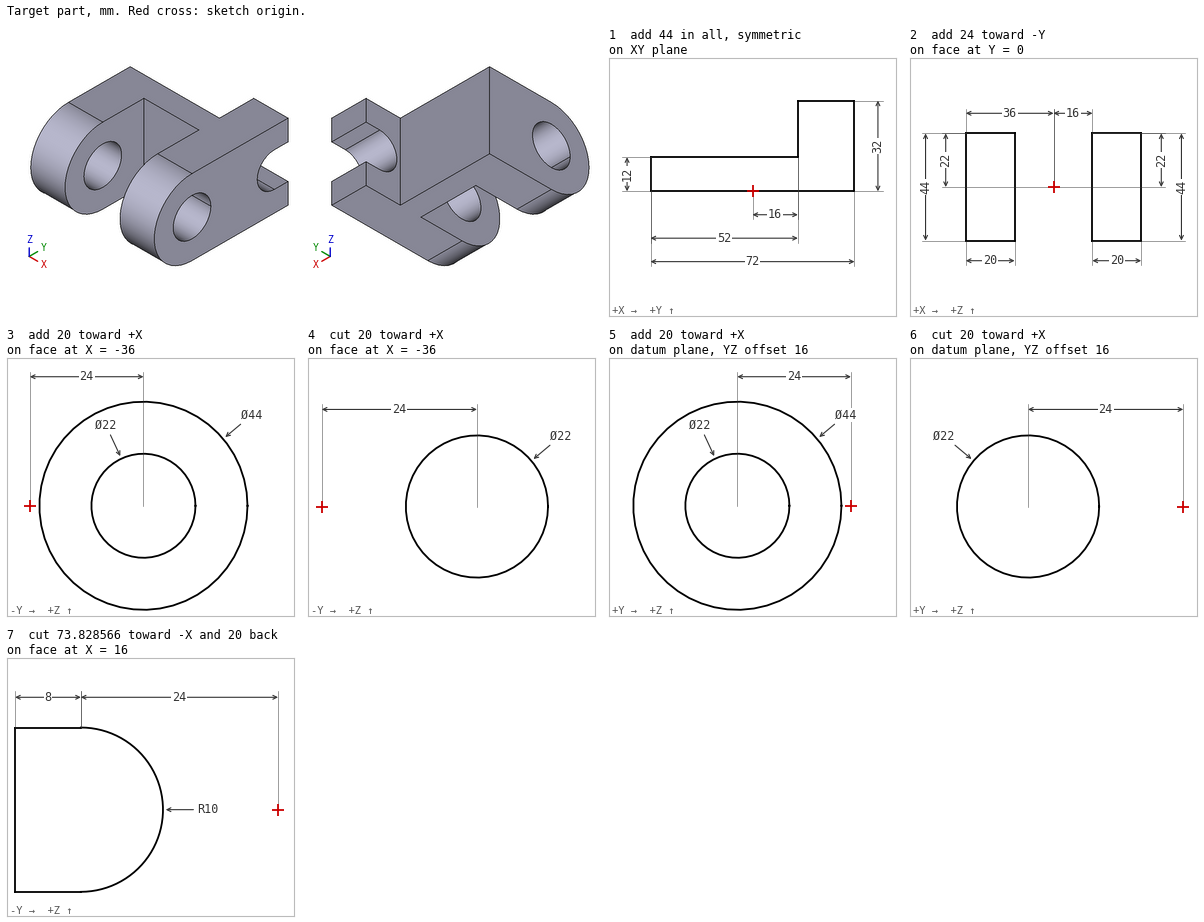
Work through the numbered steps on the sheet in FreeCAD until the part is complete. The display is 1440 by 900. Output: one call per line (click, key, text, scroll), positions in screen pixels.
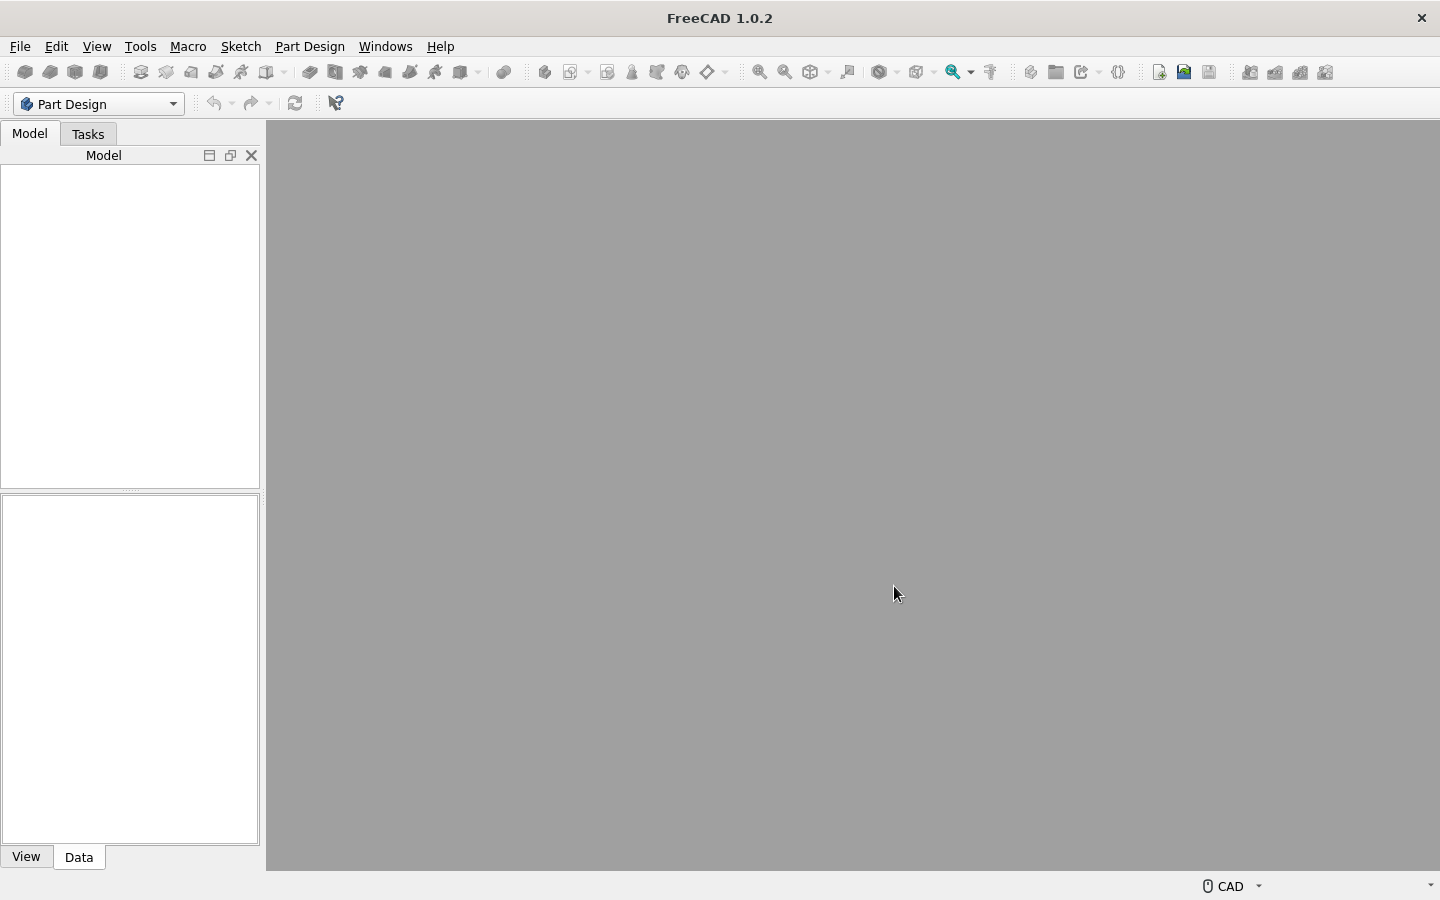
click(1159, 72)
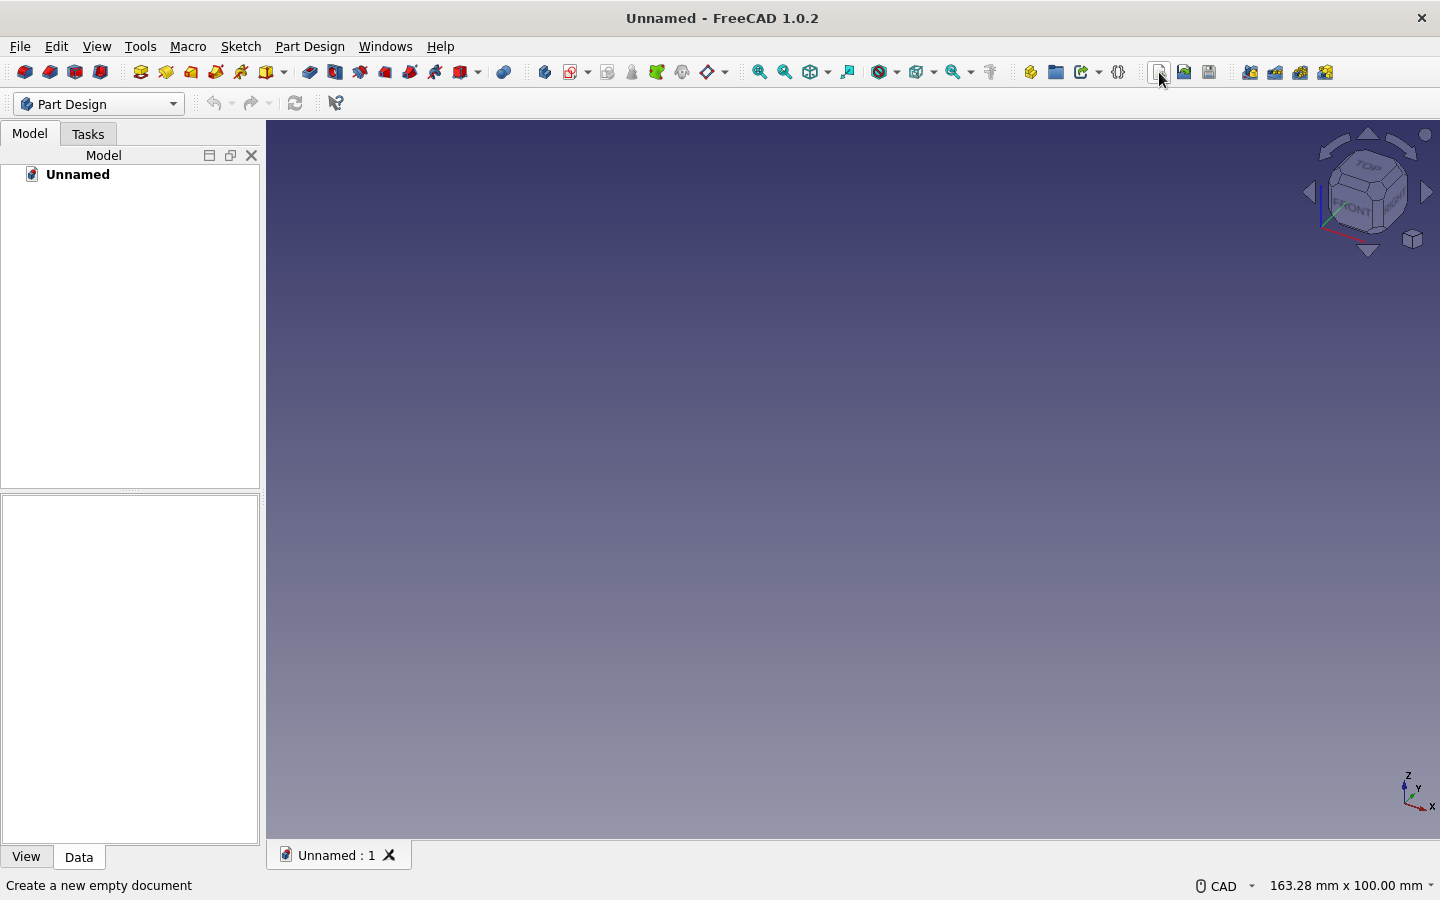
click(570, 72)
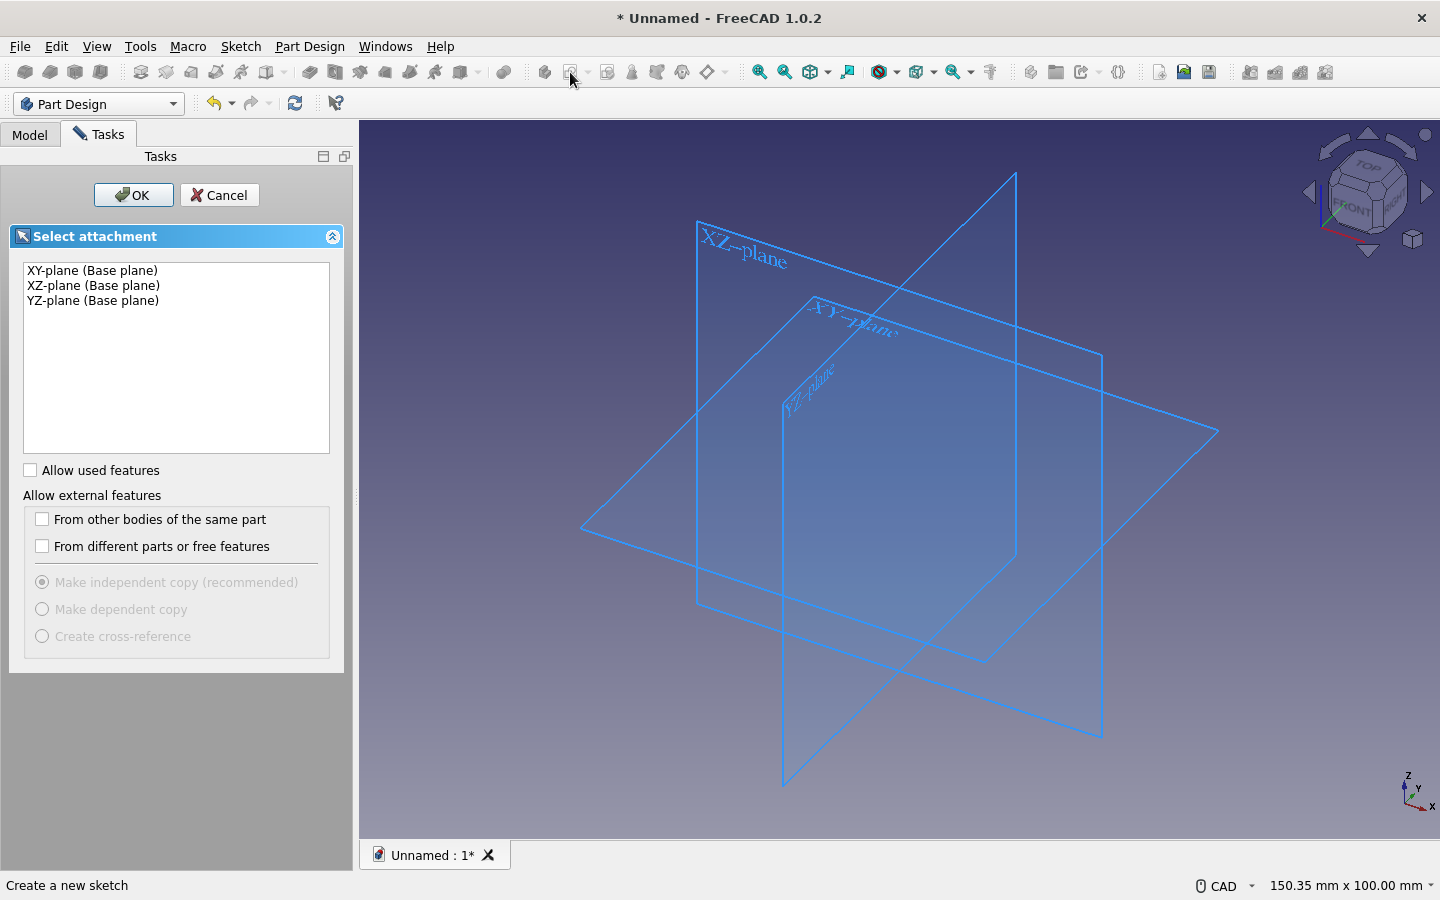
click(84, 270)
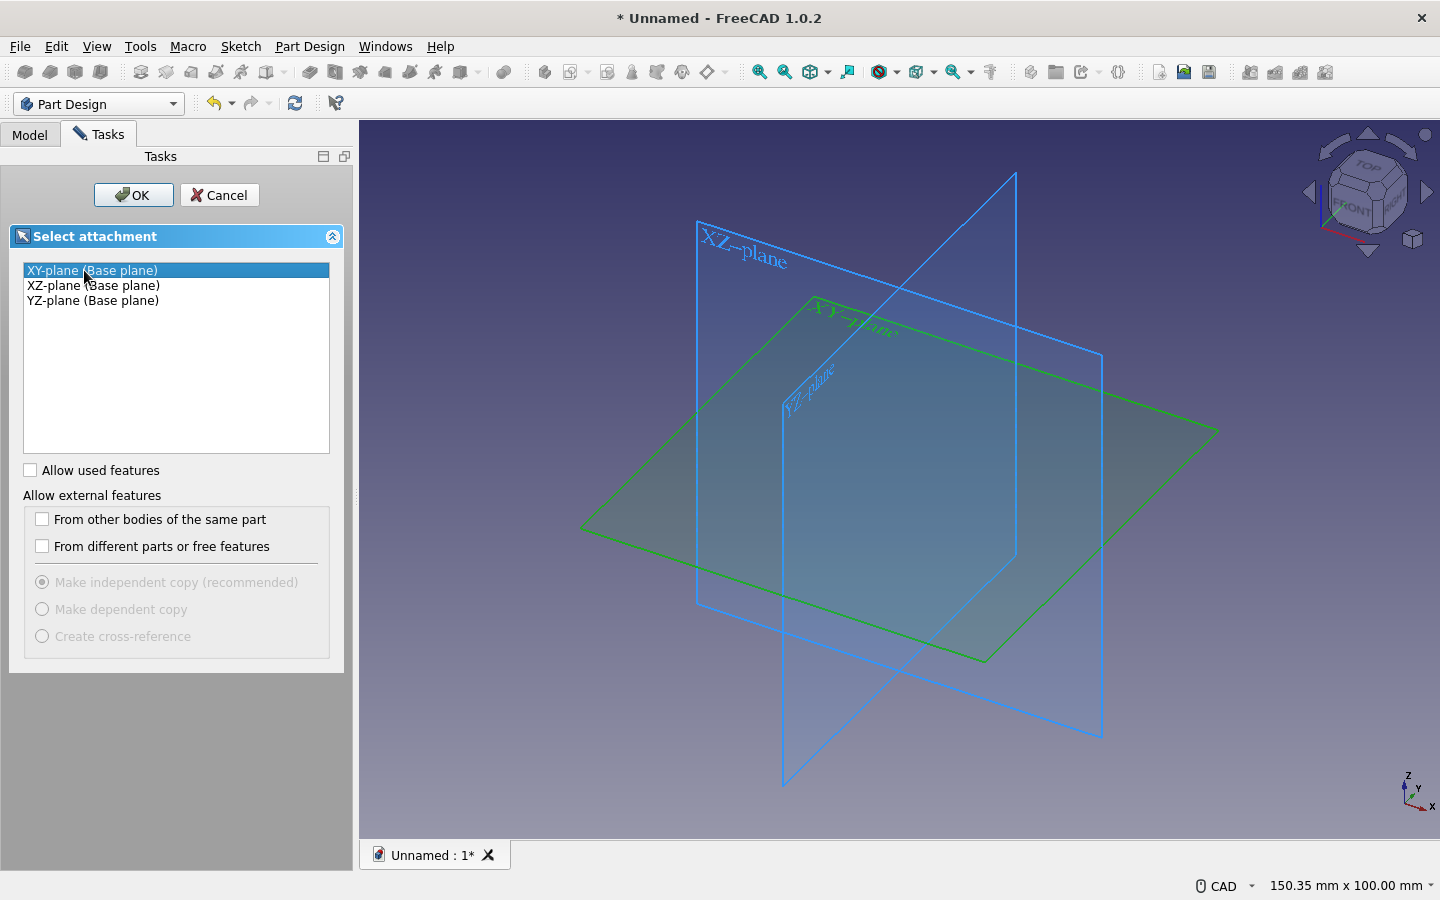
click(134, 195)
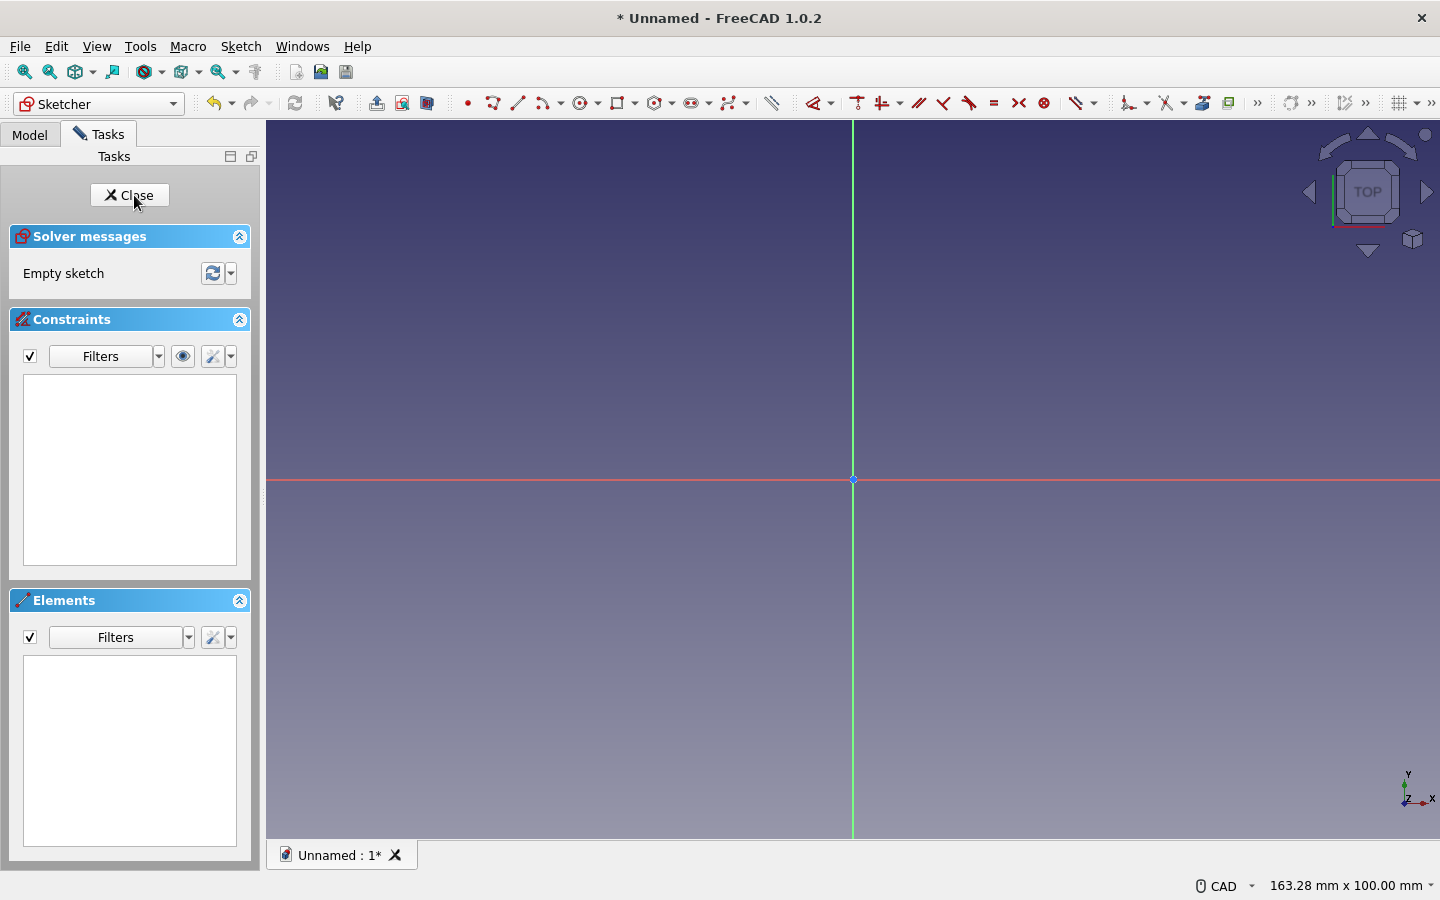
click(493, 104)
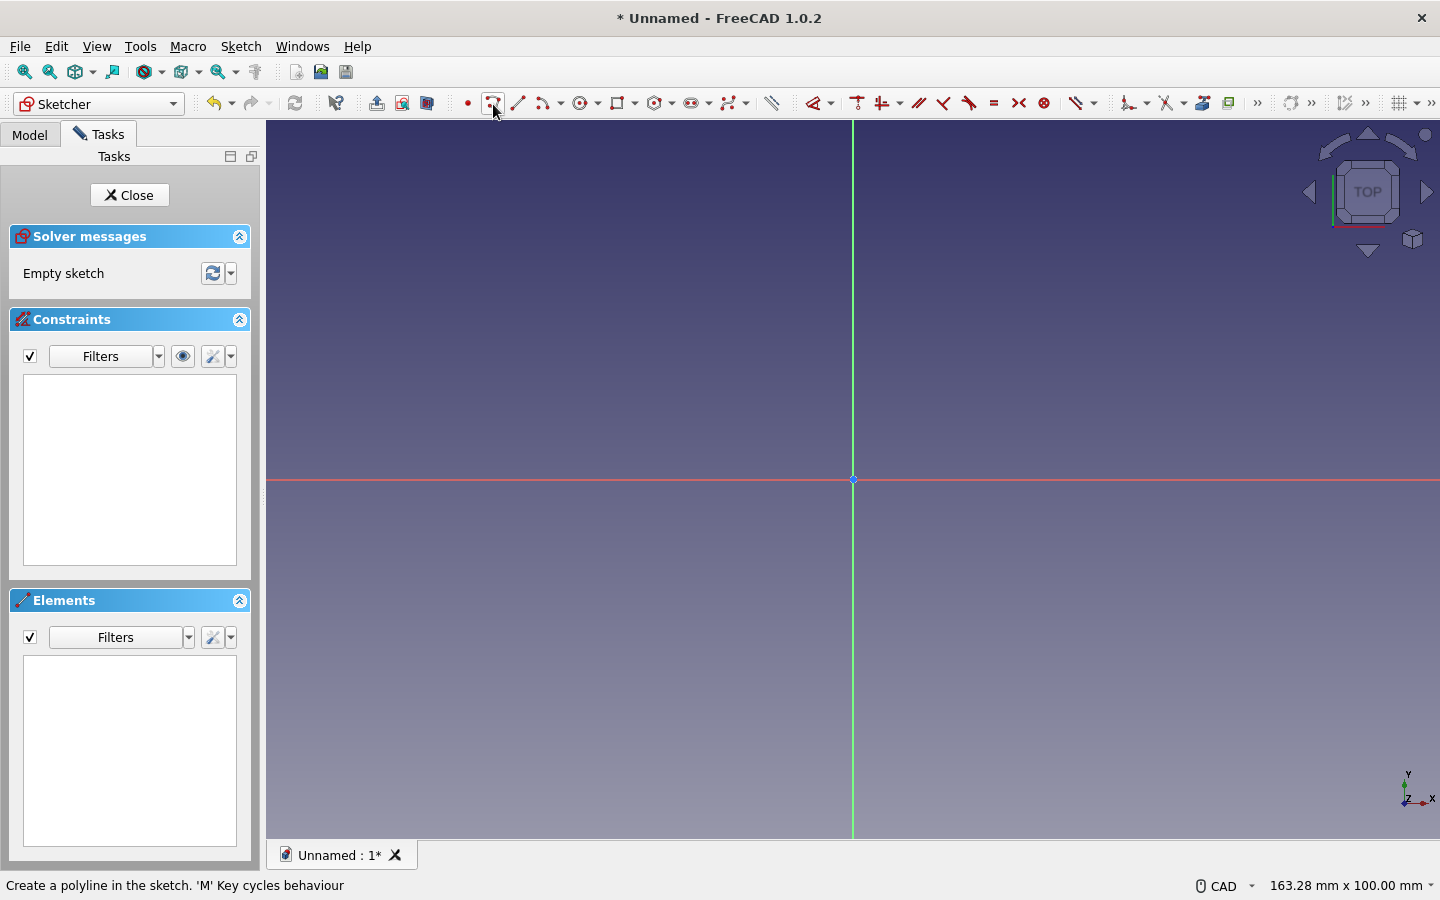
click(968, 393)
click(594, 393)
click(594, 480)
click(1112, 470)
click(1112, 249)
click(968, 249)
click(968, 394)
key(Escape)
key(Escape)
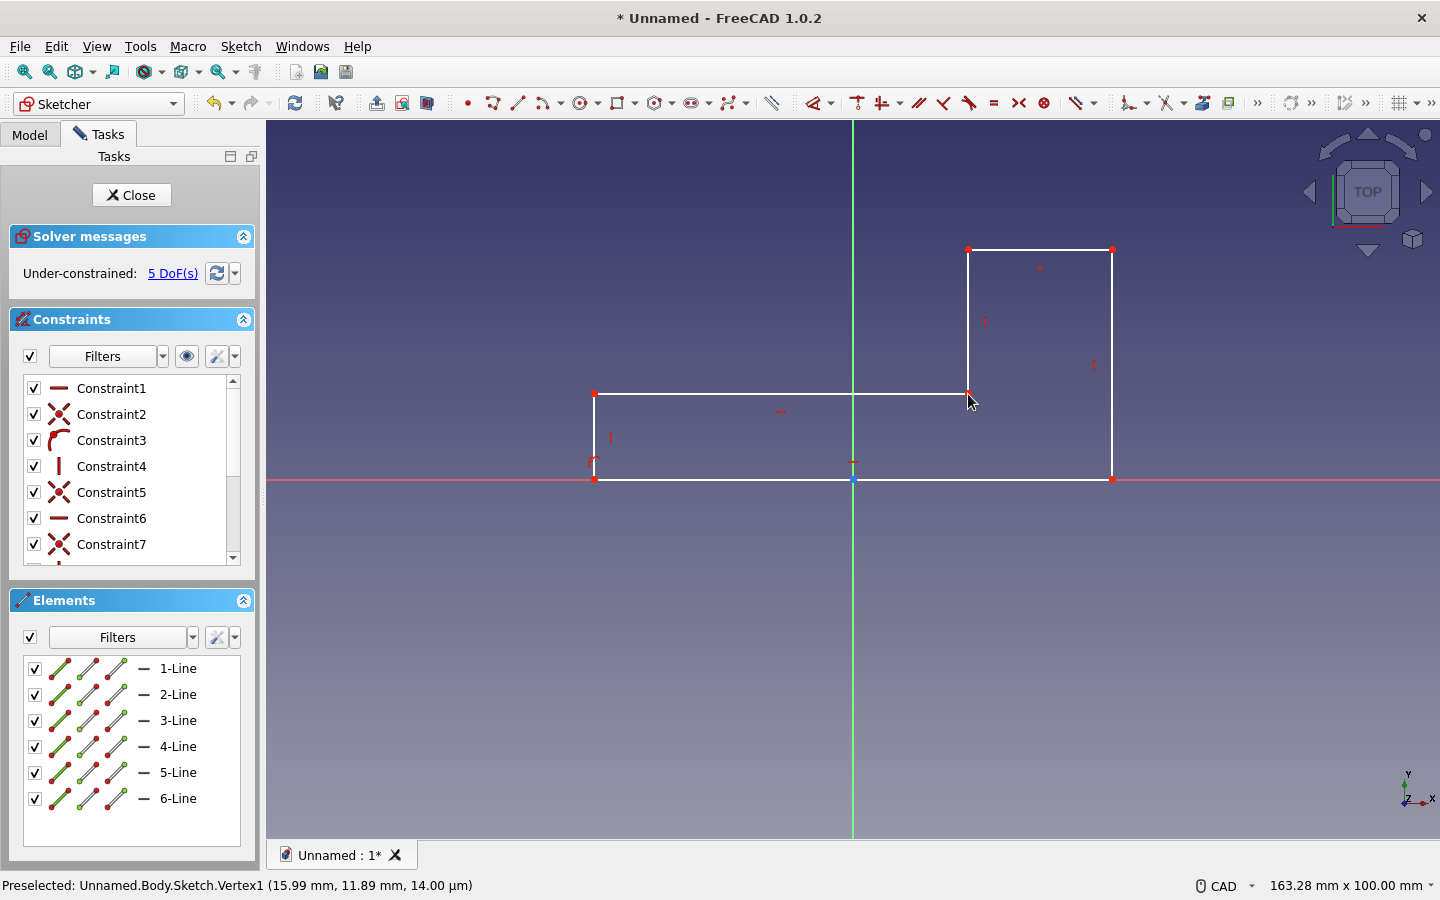
click(812, 104)